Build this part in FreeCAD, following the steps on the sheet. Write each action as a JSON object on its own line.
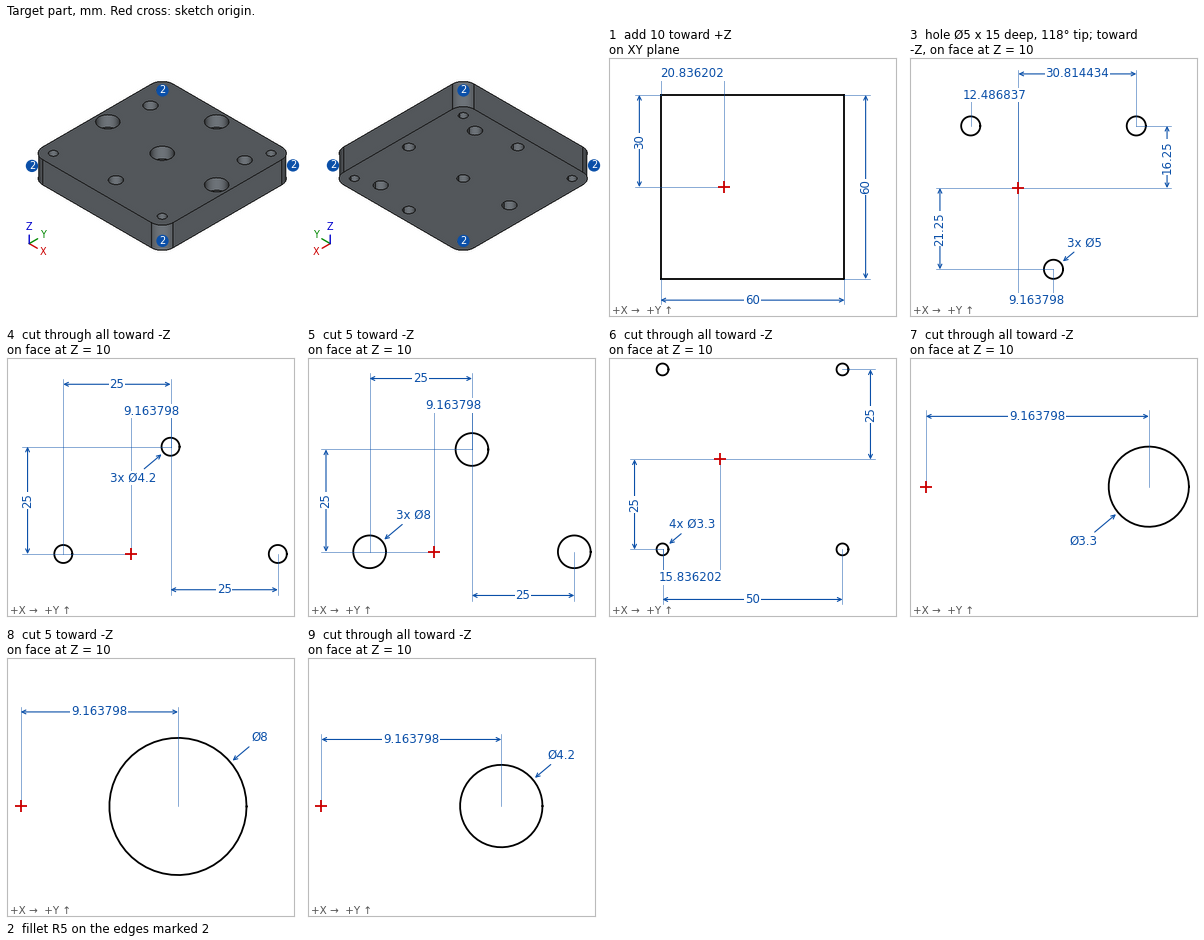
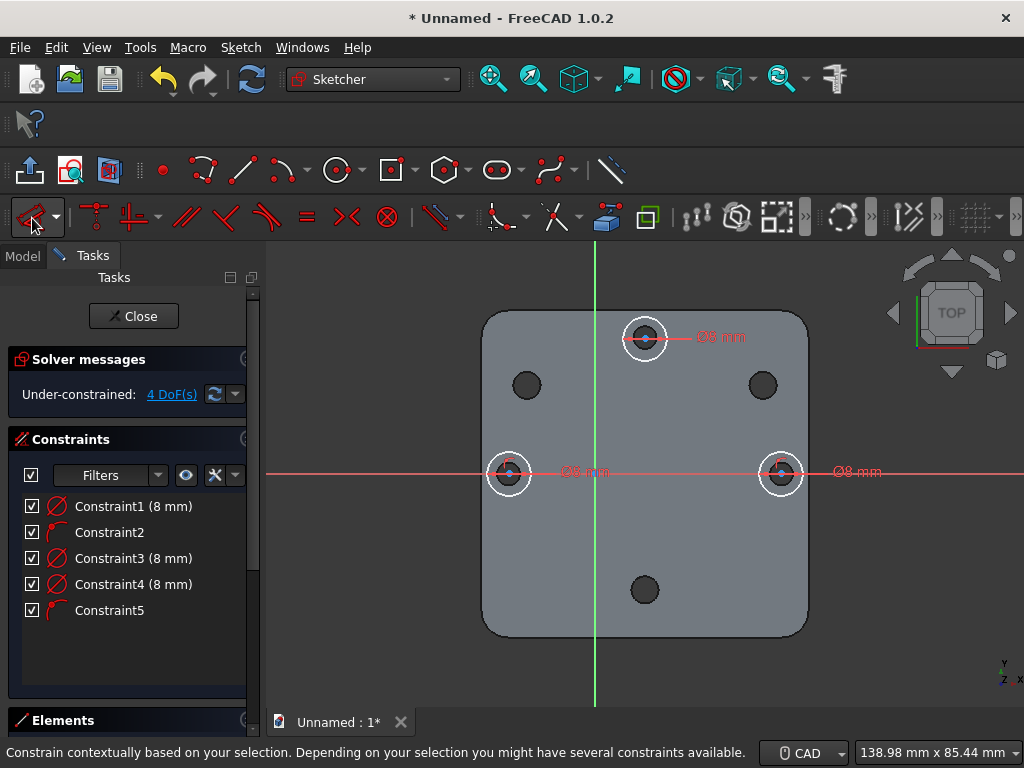
{"action": "left_click", "coordinate": [645, 339]}
{"action": "left_click", "coordinate": [561, 406]}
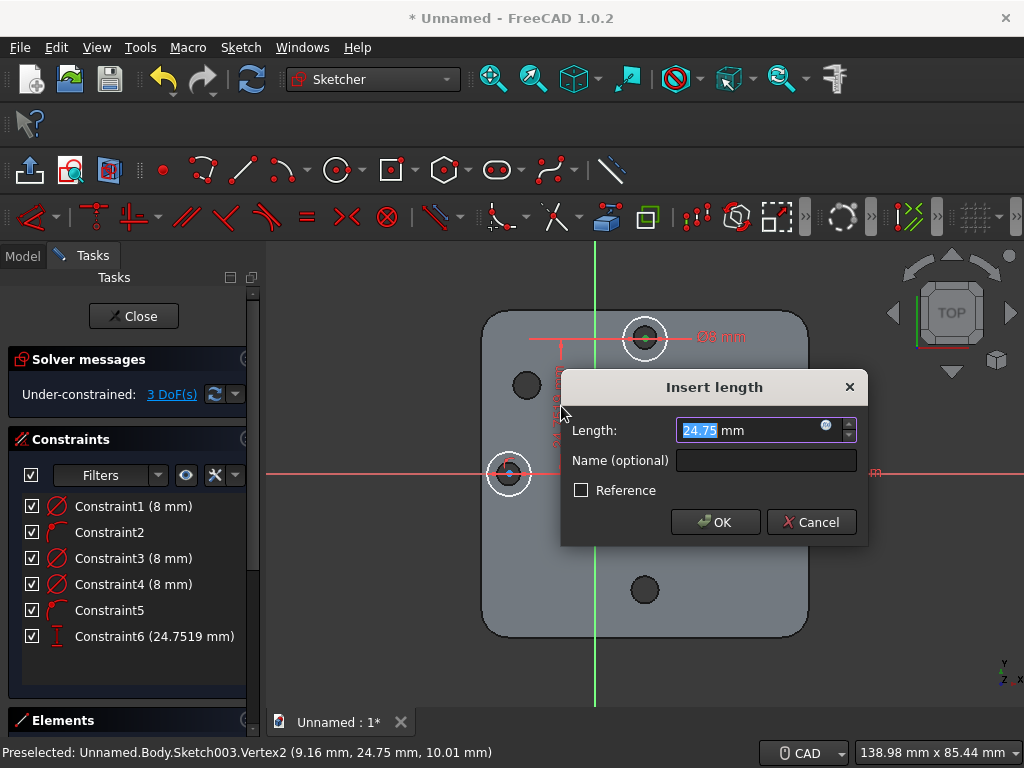
{"action": "type", "text": "25"}
{"action": "key", "text": "Return"}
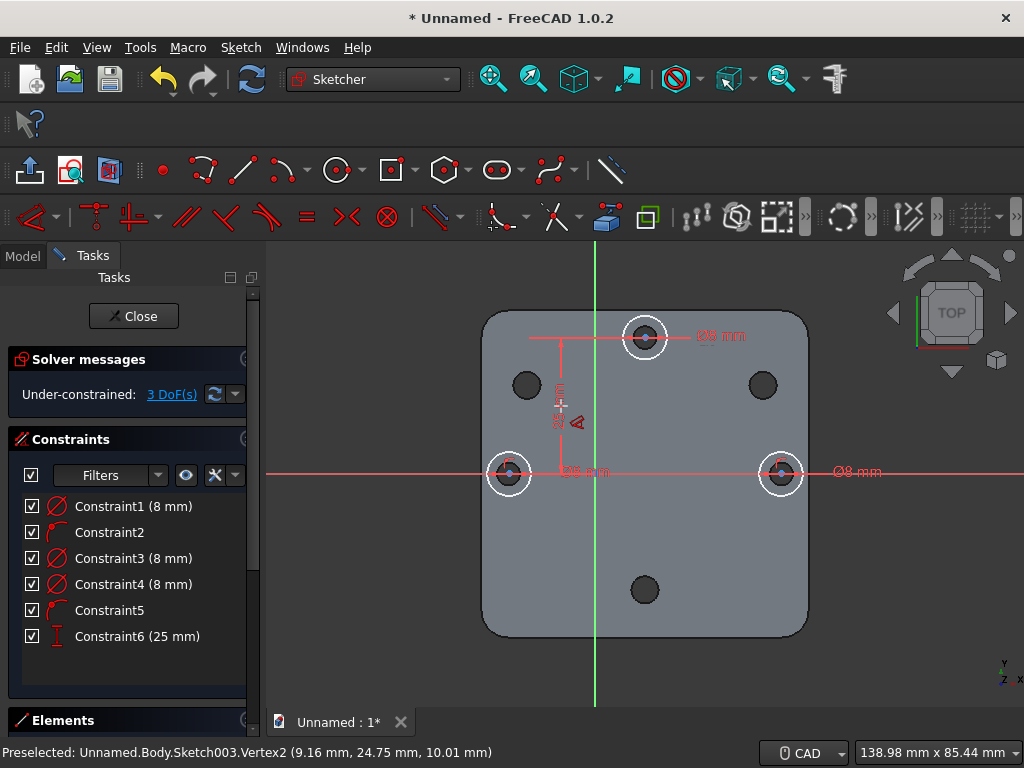
{"action": "left_click", "coordinate": [509, 474]}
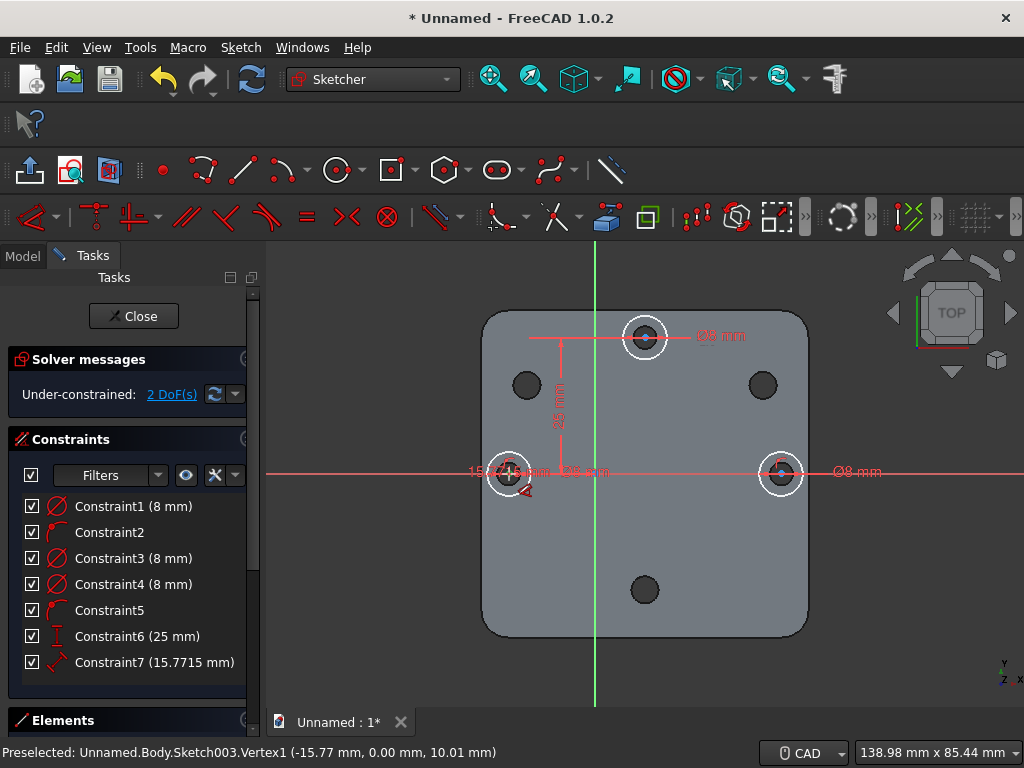
{"action": "left_click", "coordinate": [645, 338]}
{"action": "left_click", "coordinate": [577, 508]}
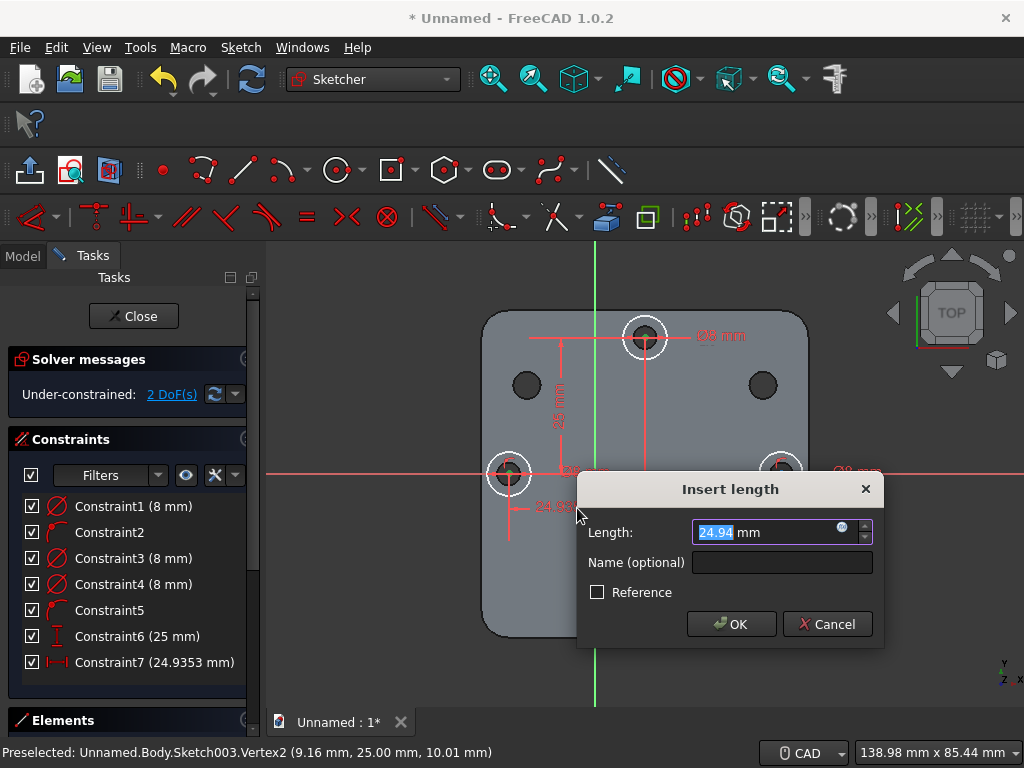
{"action": "type", "text": "25"}
{"action": "key", "text": "Return"}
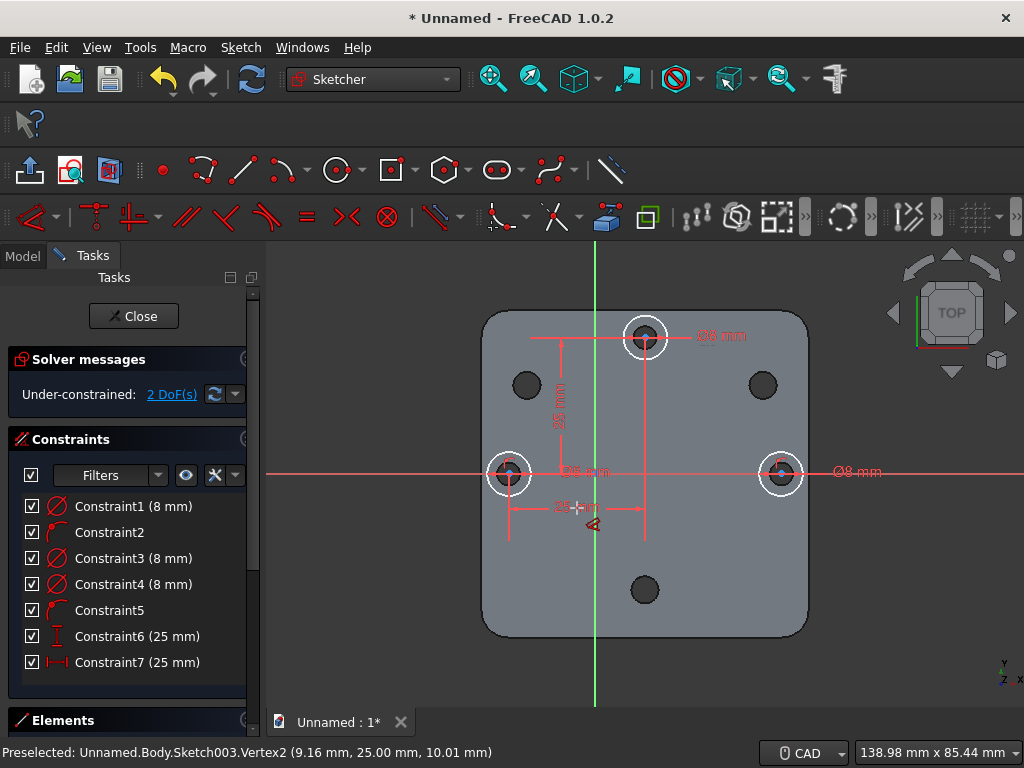
{"action": "left_click", "coordinate": [645, 338]}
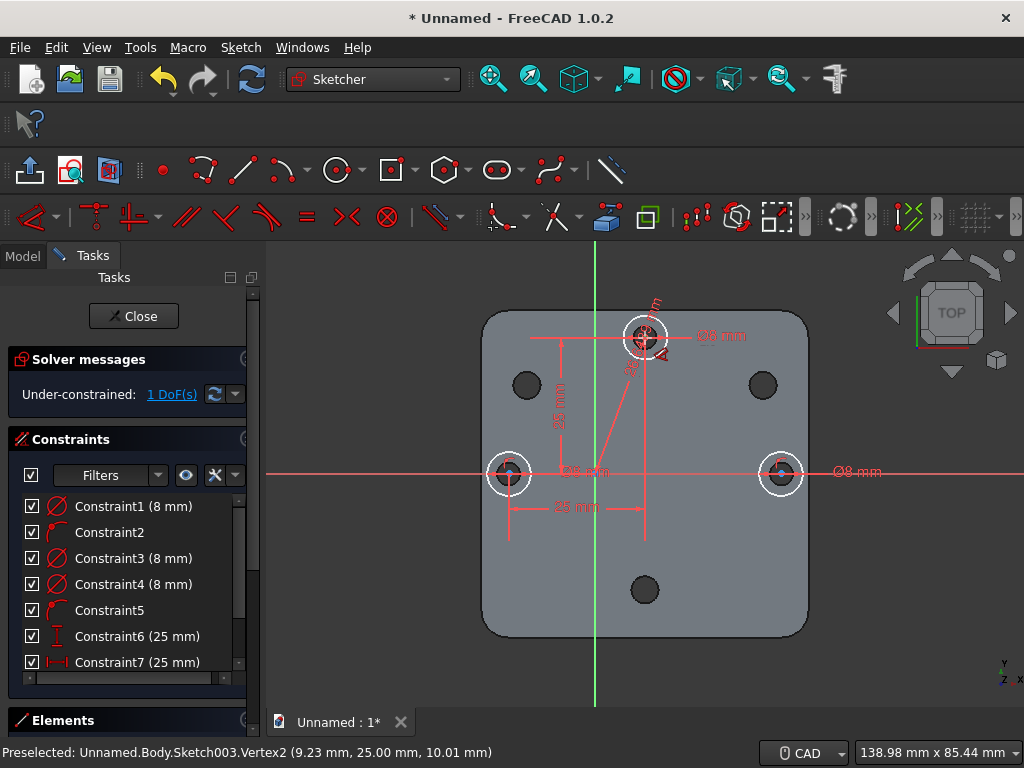
{"action": "left_click", "coordinate": [781, 474]}
{"action": "left_click", "coordinate": [713, 508]}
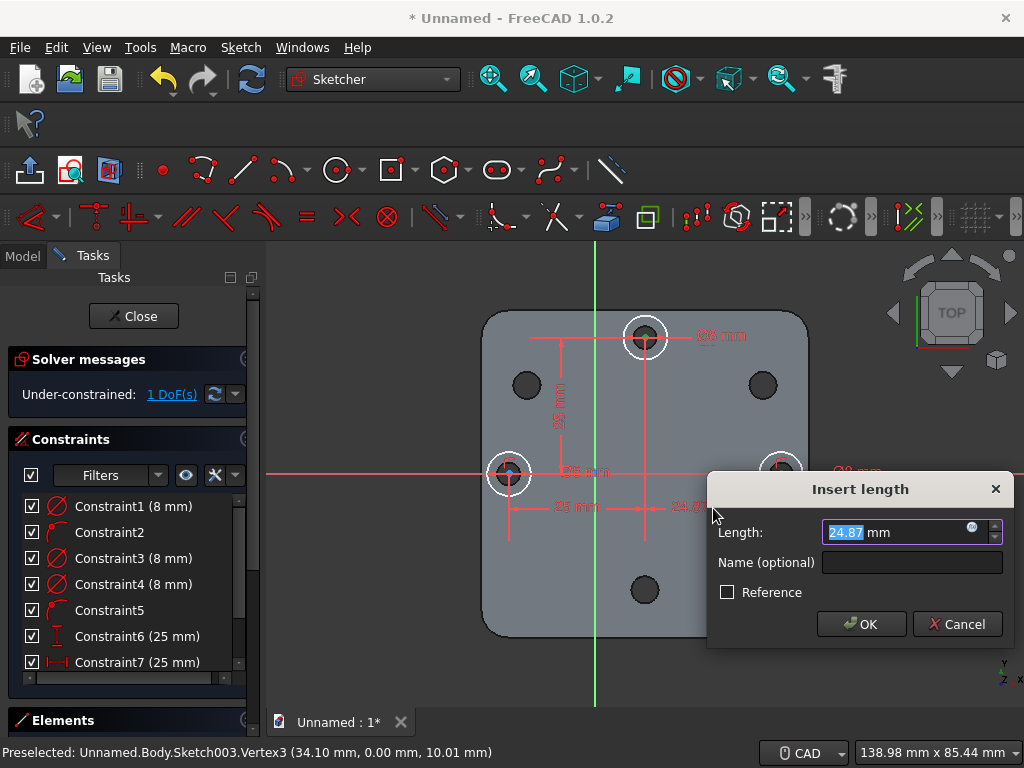
{"action": "type", "text": "25"}
{"action": "key", "text": "Return"}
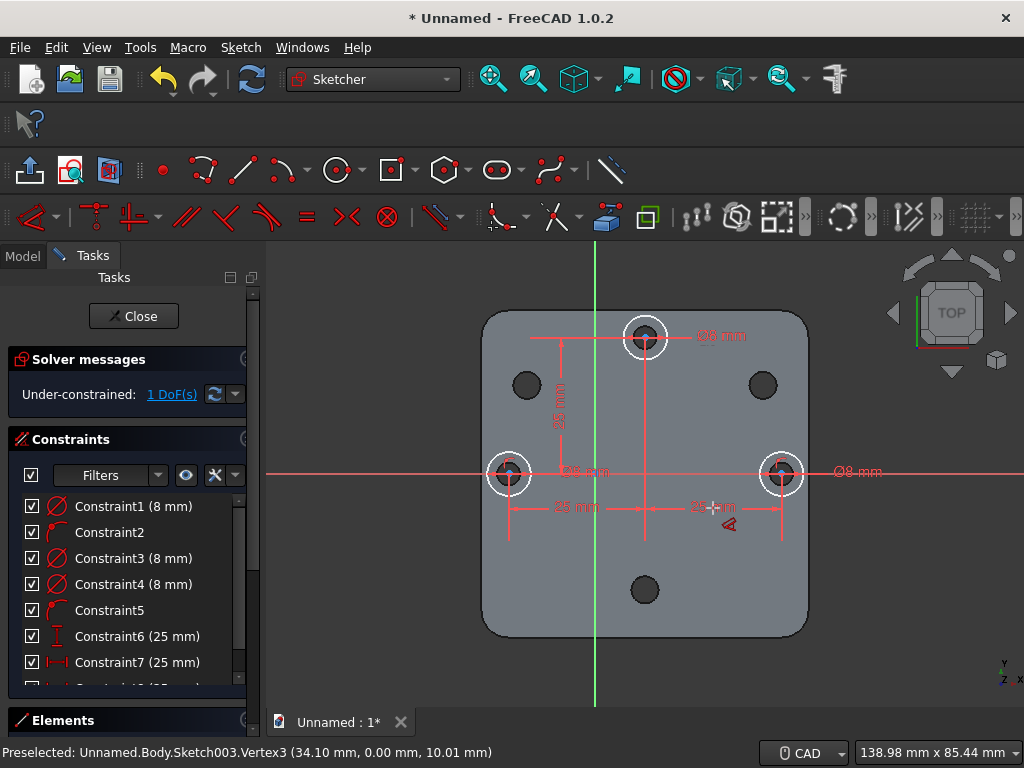
{"action": "left_click", "coordinate": [645, 338]}
{"action": "left_click", "coordinate": [620, 304]}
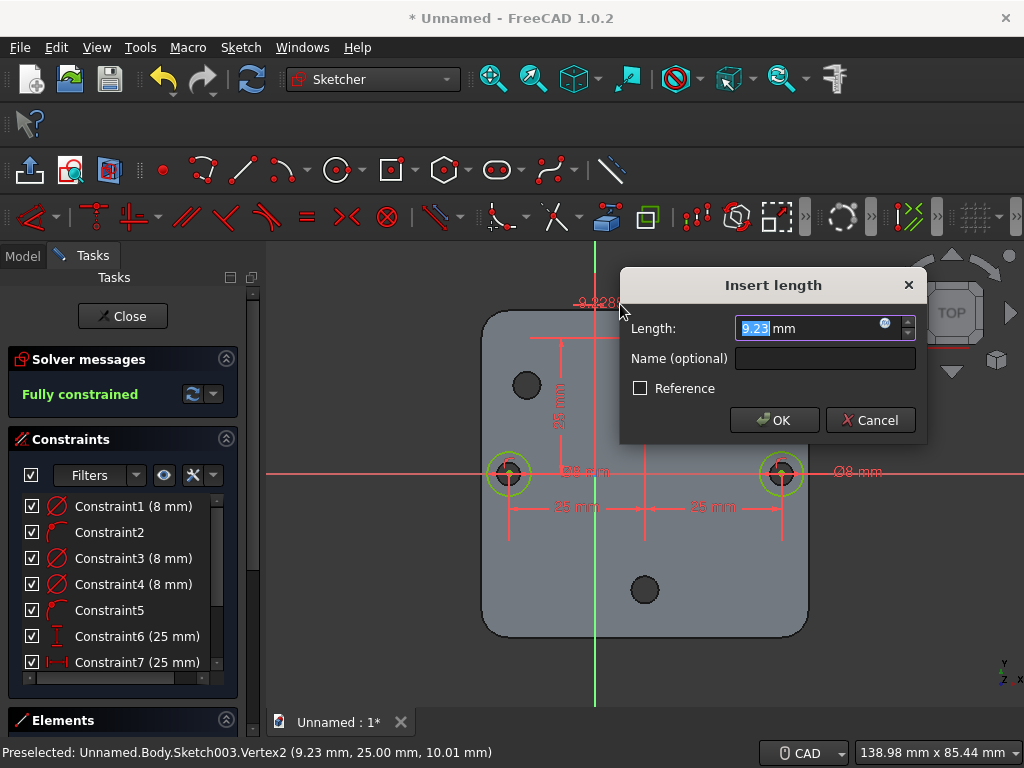
{"action": "type", "text": "9.163798"}
{"action": "key", "text": "Return"}
{"action": "key", "text": "Escape"}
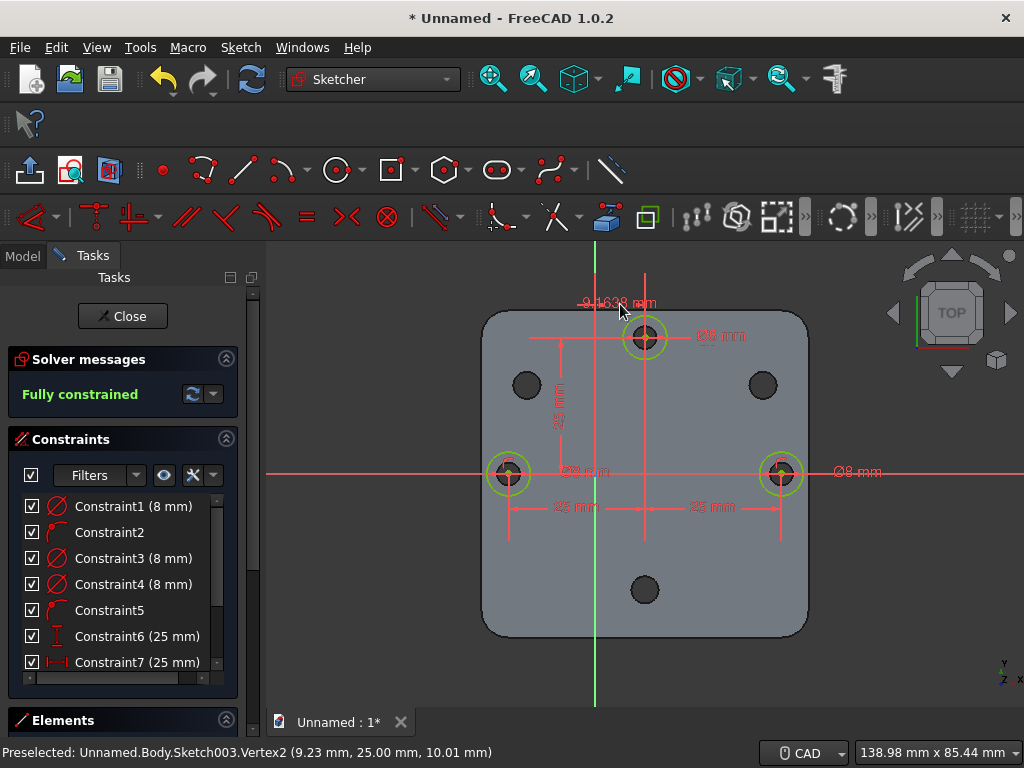
{"action": "left_click", "coordinate": [123, 316]}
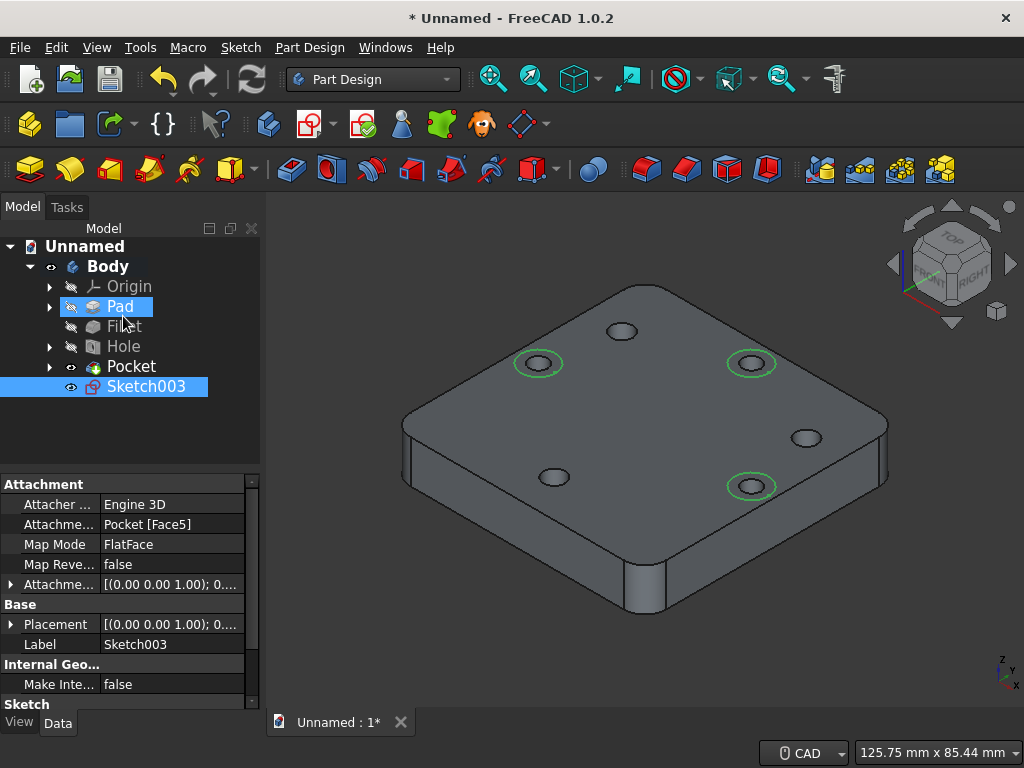
{"action": "left_click", "coordinate": [292, 170]}